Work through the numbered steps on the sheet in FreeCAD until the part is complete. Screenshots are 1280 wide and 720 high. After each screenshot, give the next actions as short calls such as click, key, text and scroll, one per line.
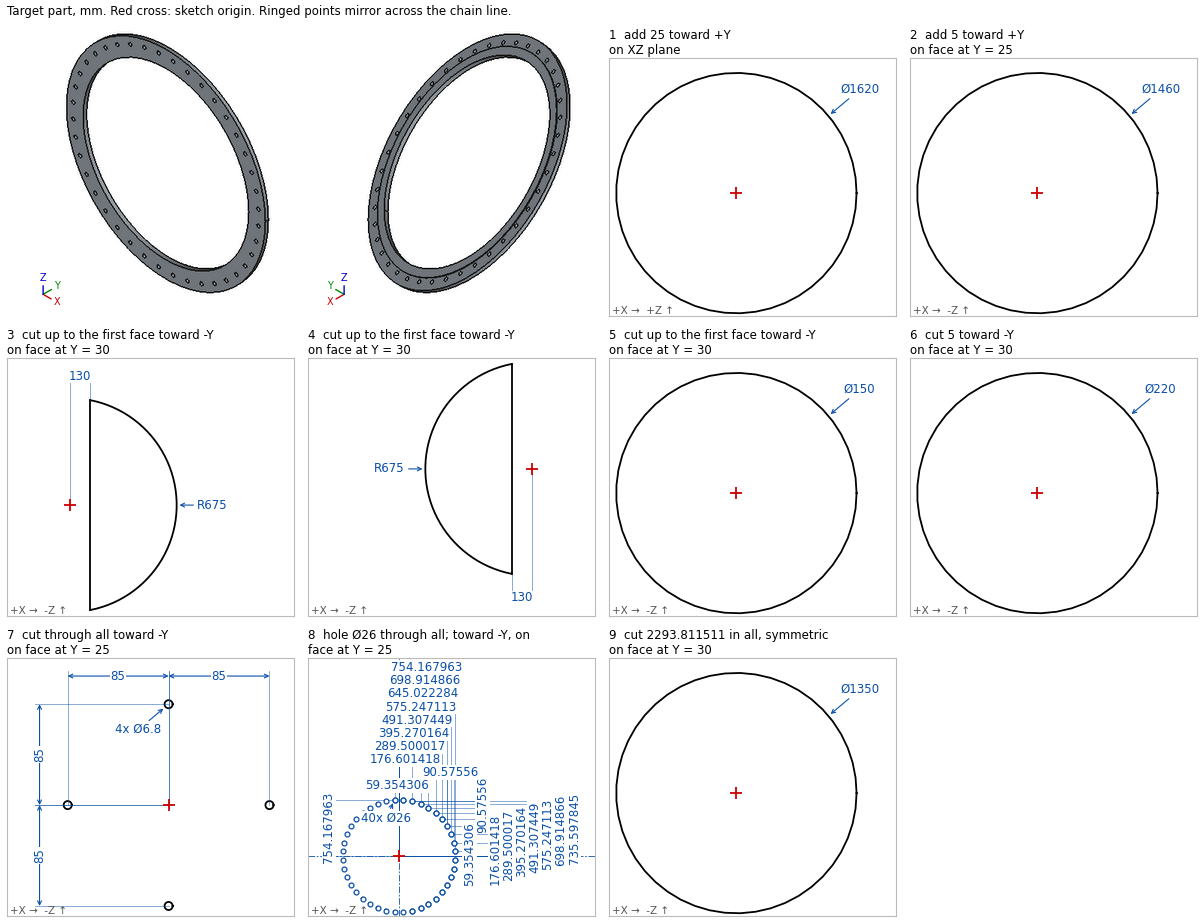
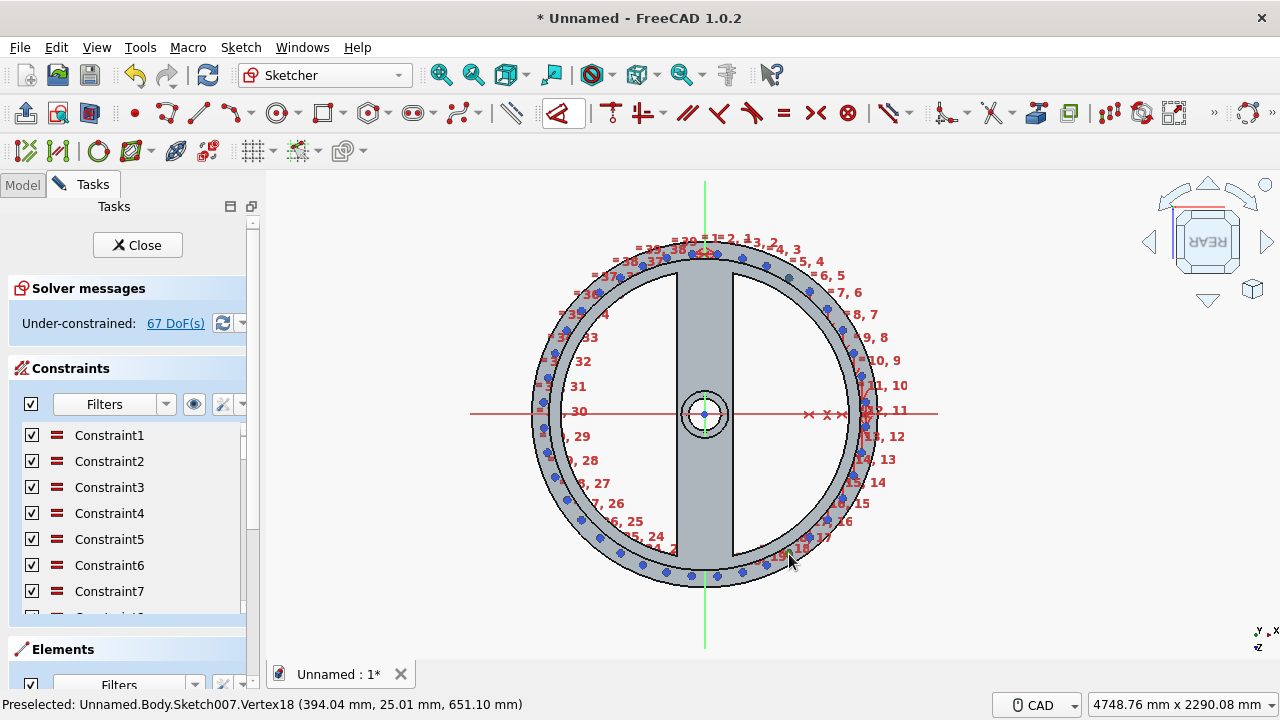
click(470, 414)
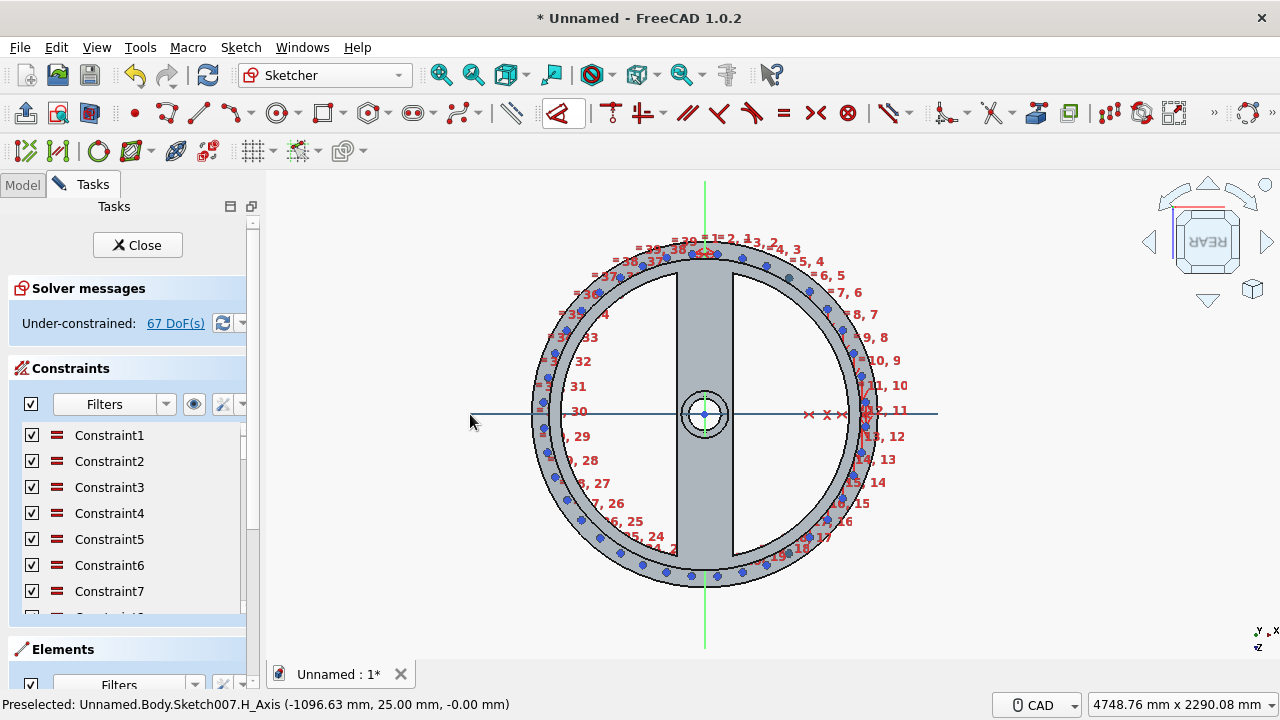
key(s)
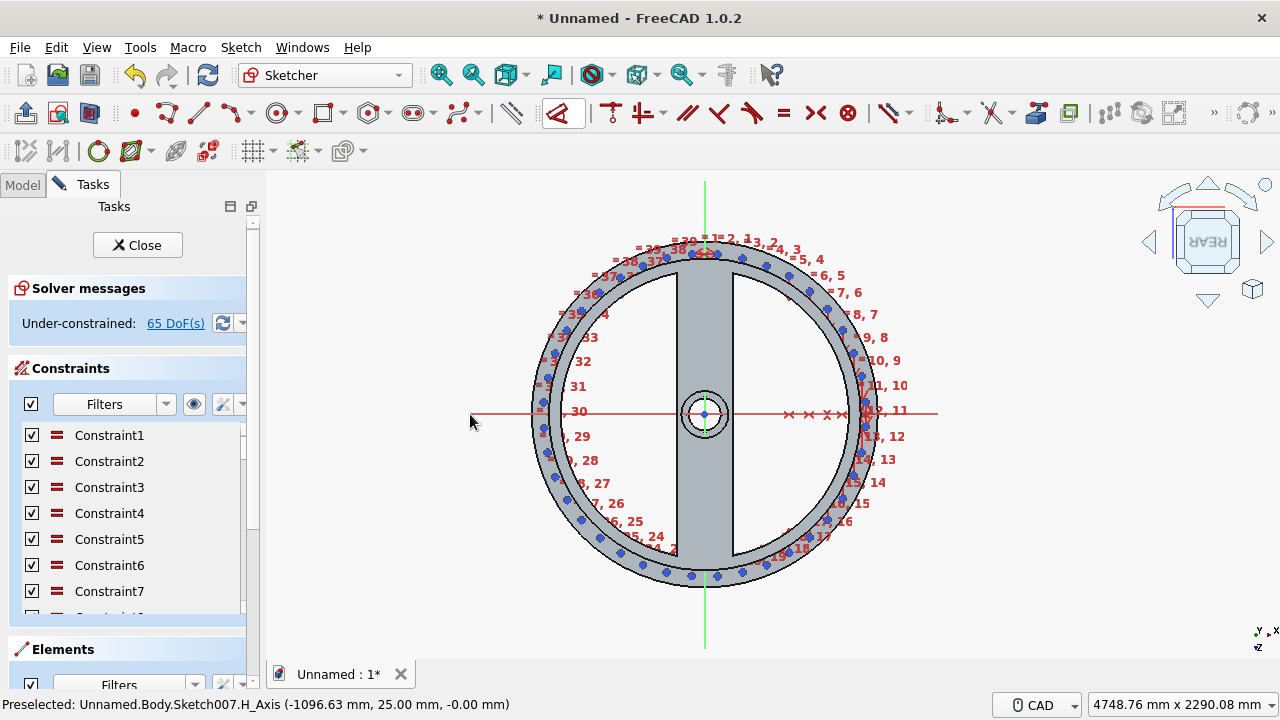
click(767, 266)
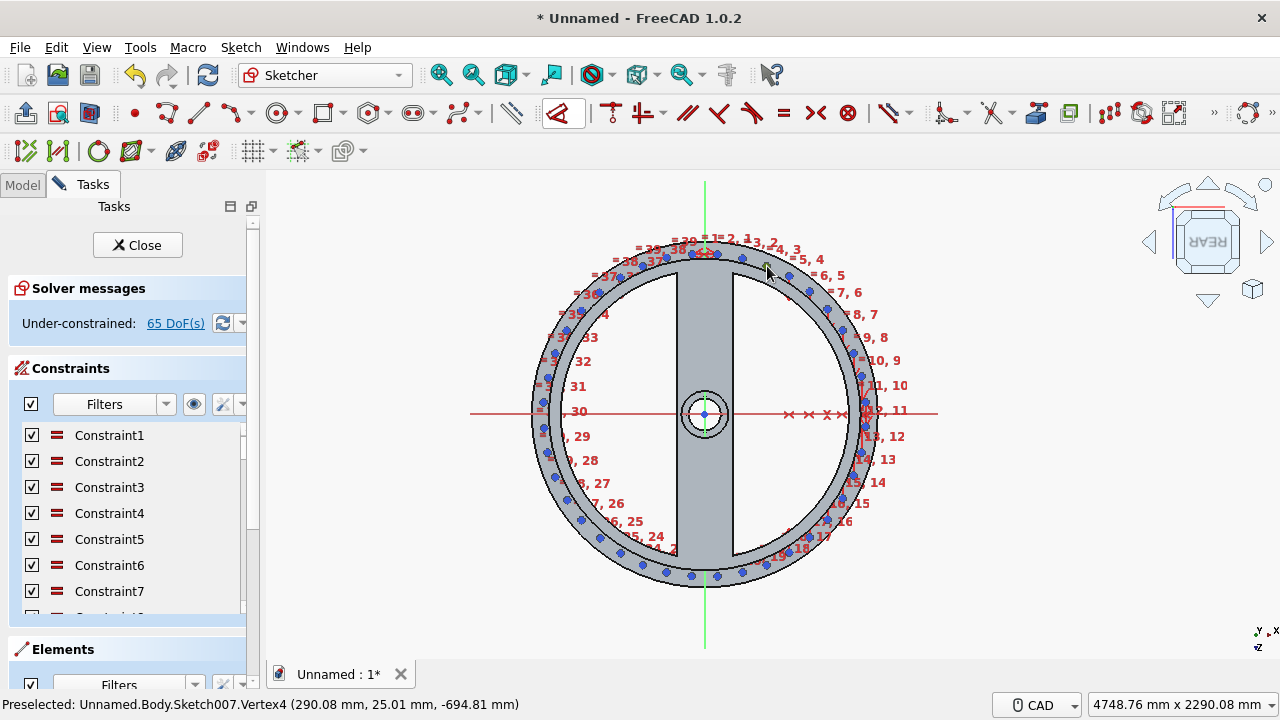
click(767, 565)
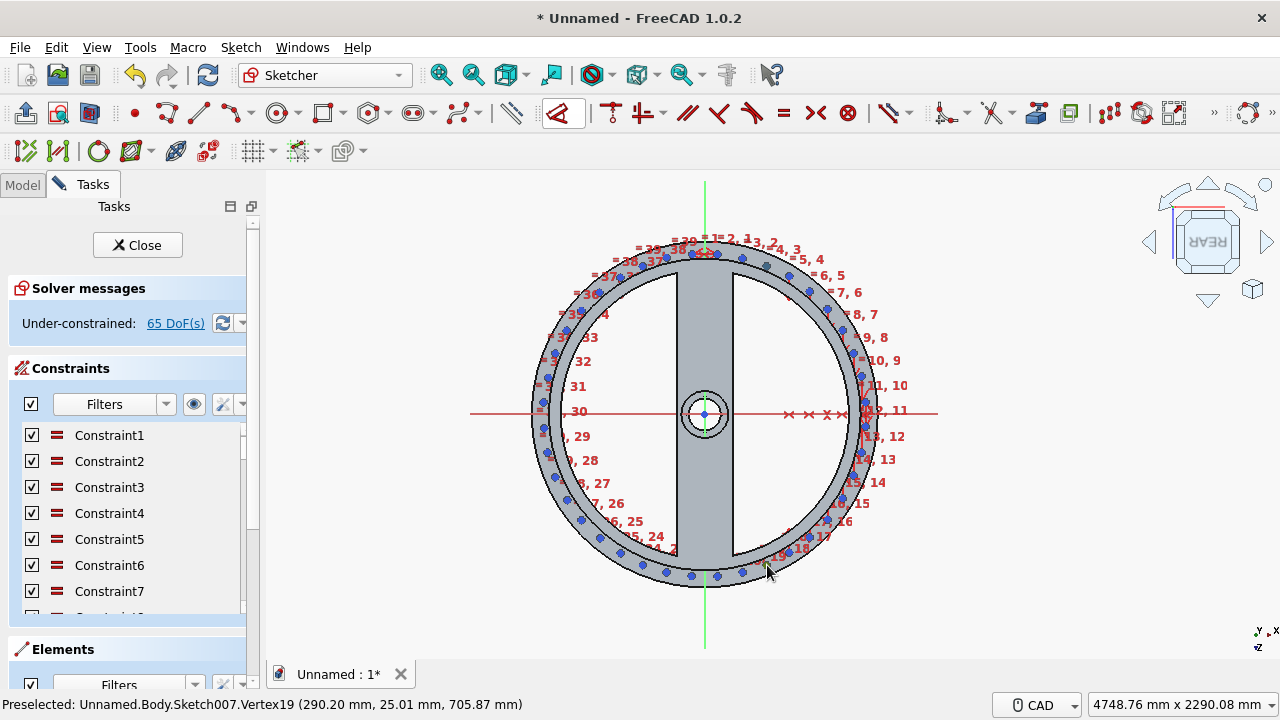
click(470, 414)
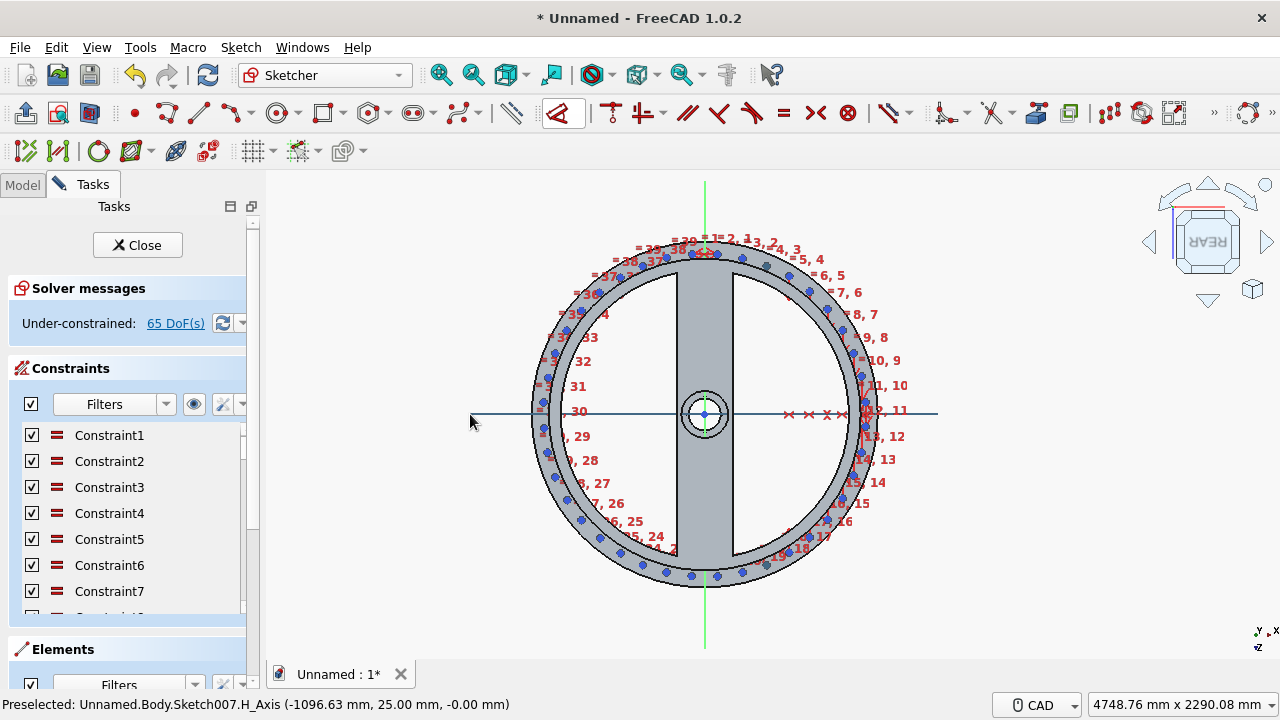
key(s)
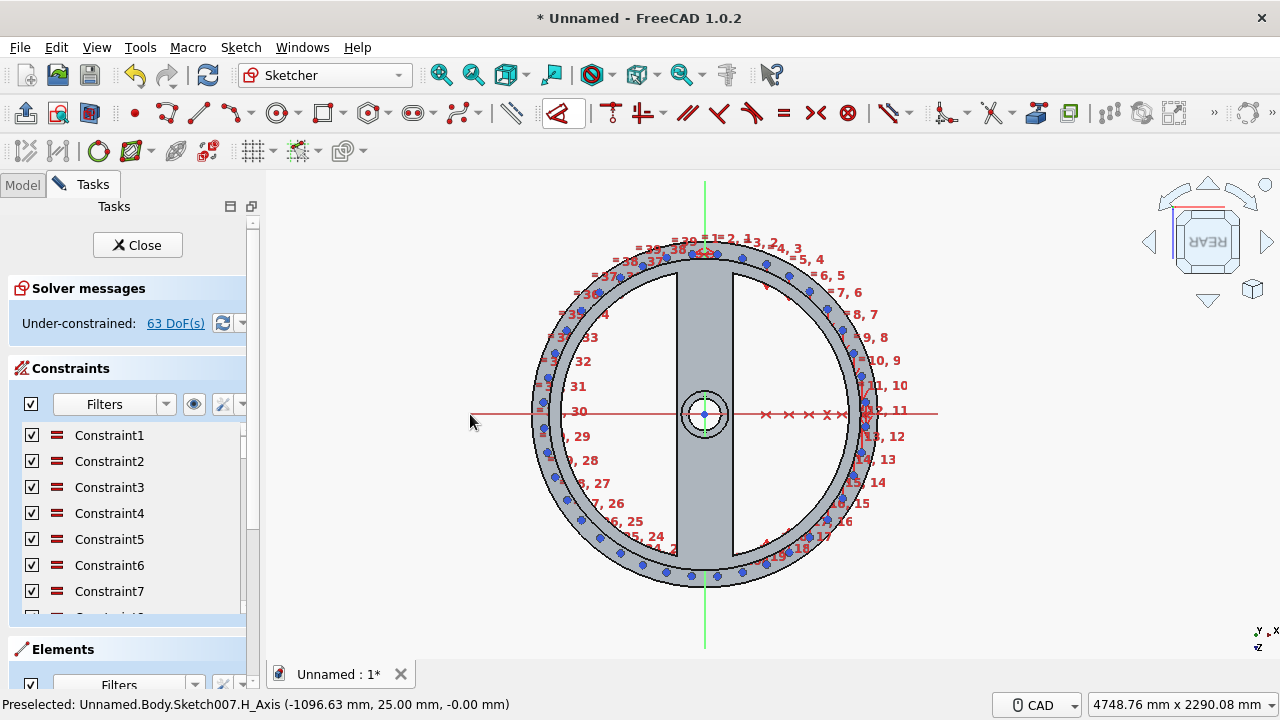
click(743, 259)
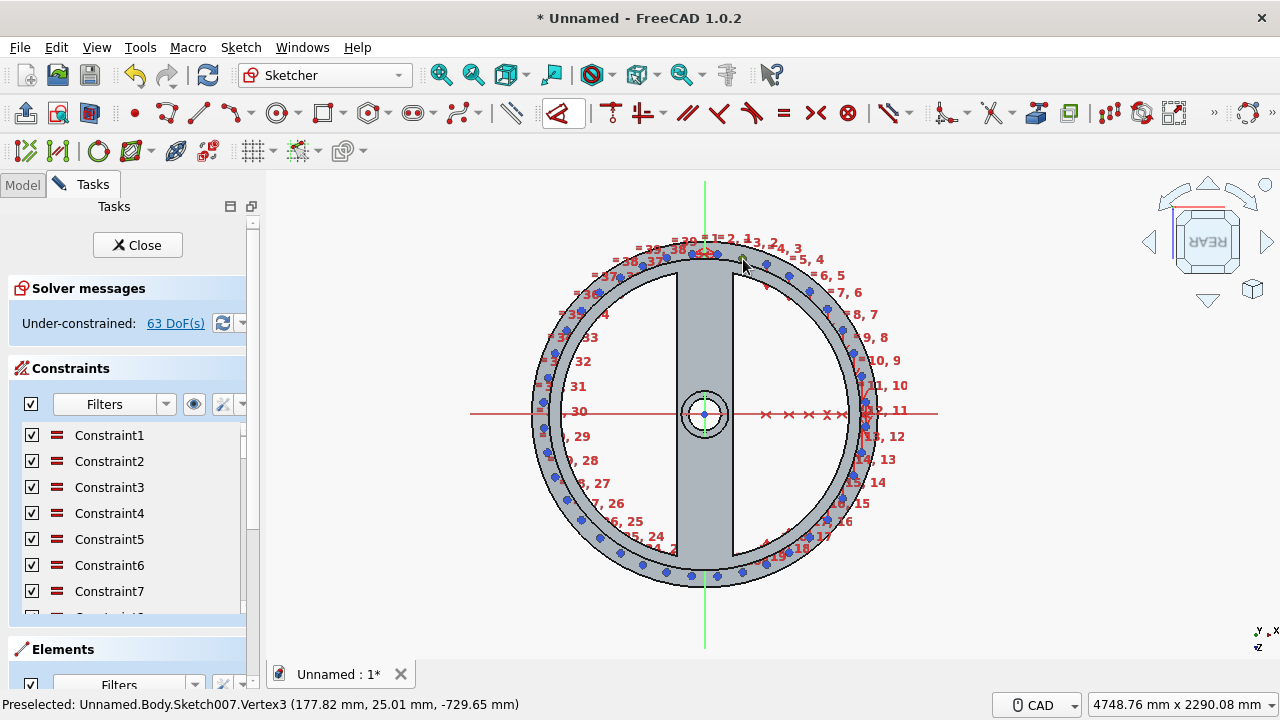
click(743, 572)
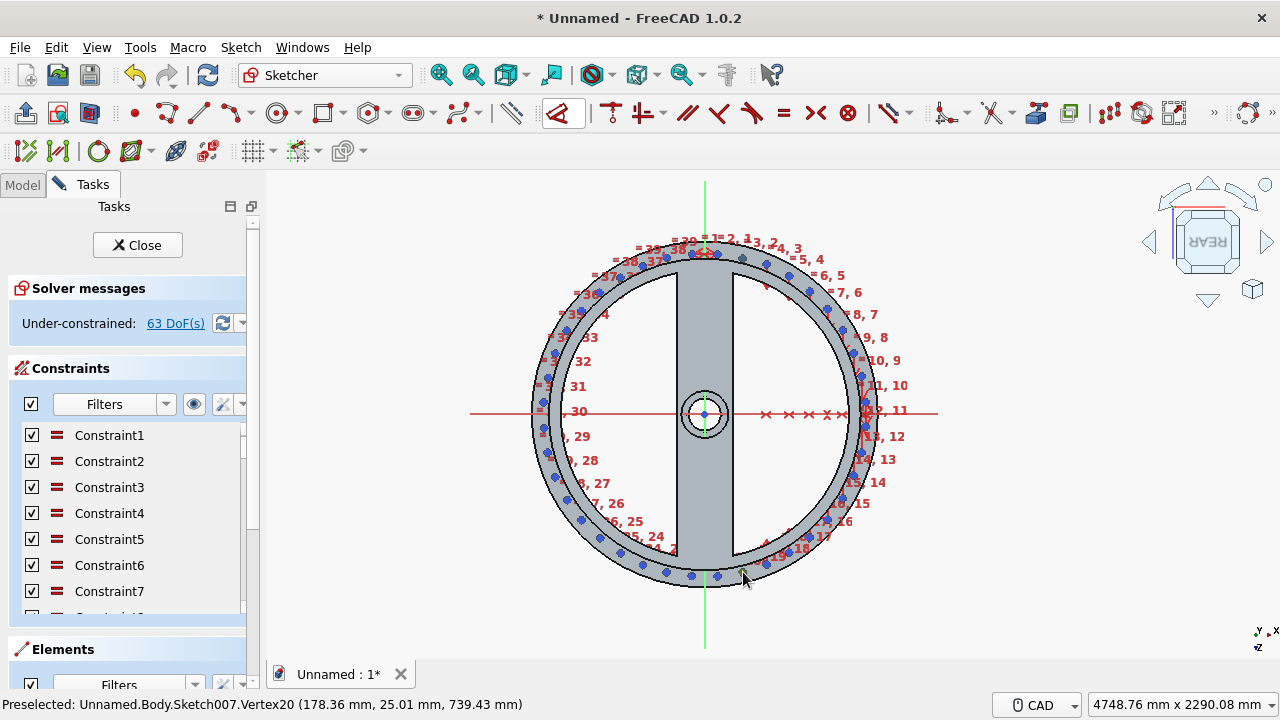
click(470, 414)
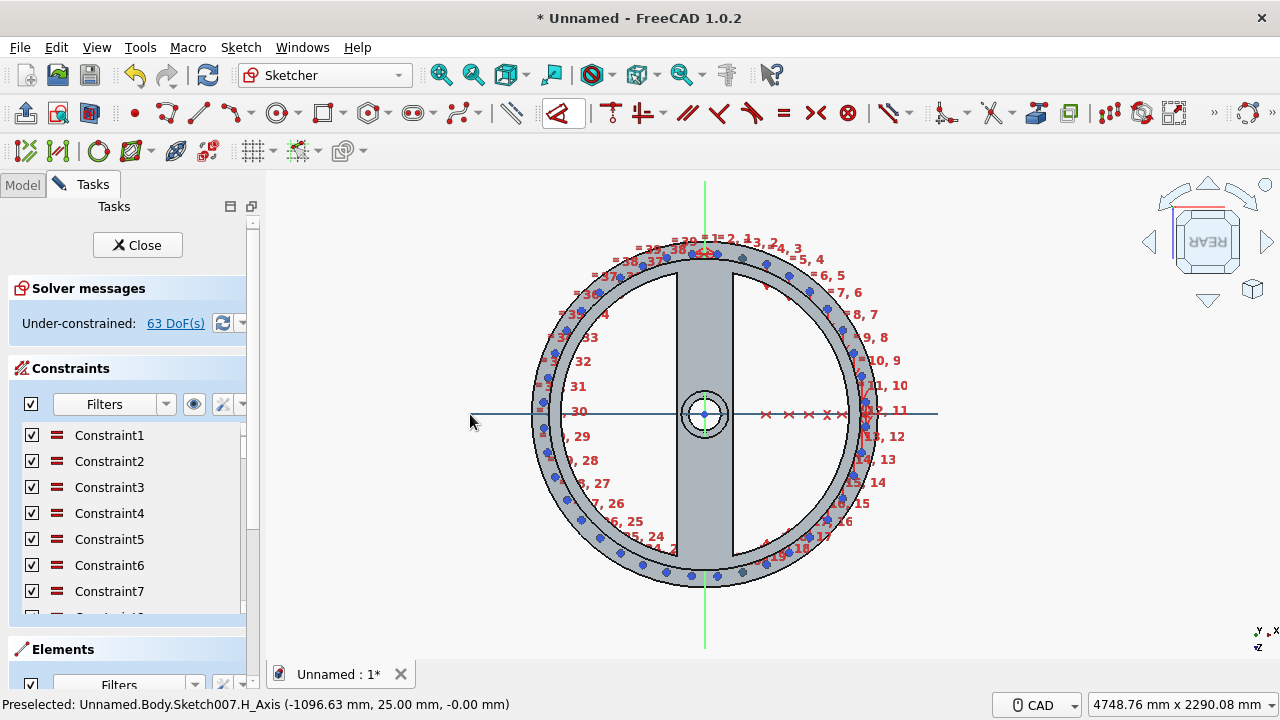
key(s)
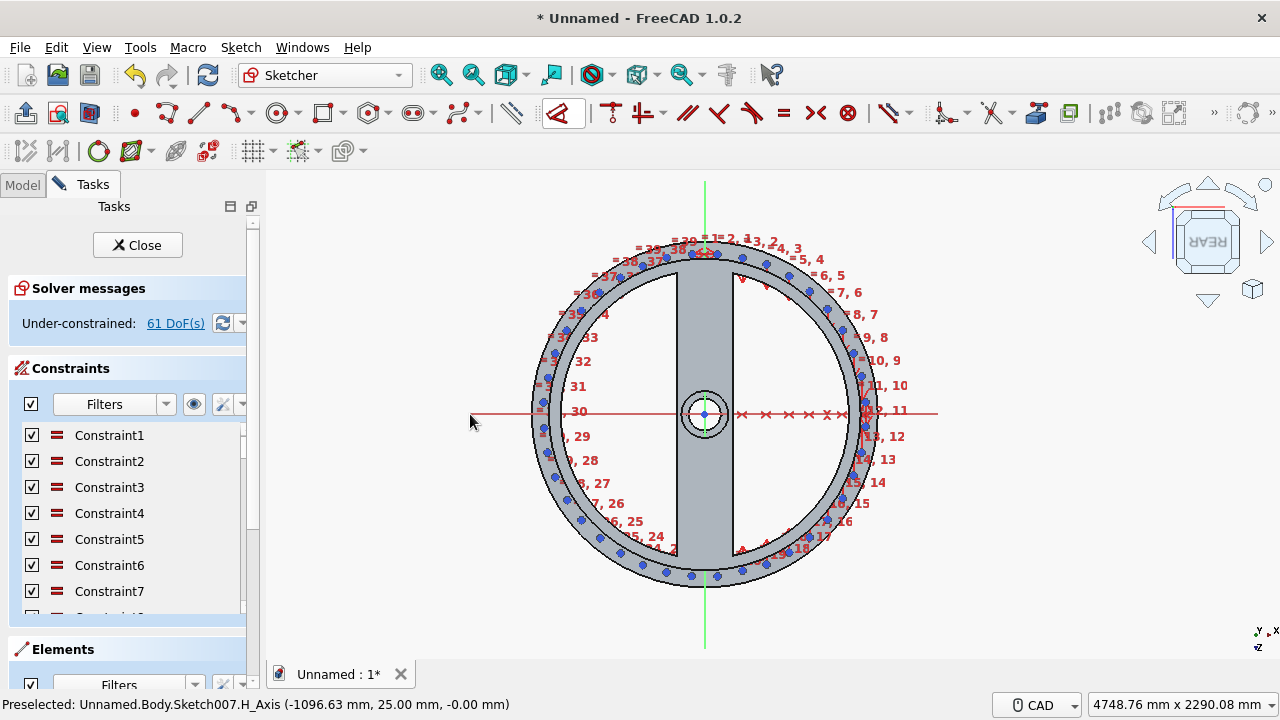
click(718, 254)